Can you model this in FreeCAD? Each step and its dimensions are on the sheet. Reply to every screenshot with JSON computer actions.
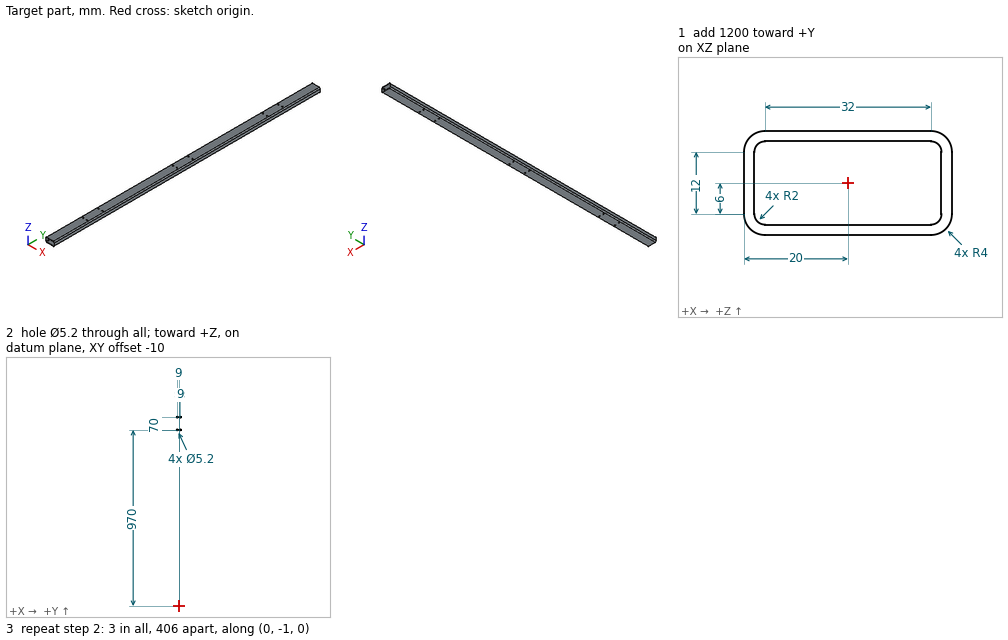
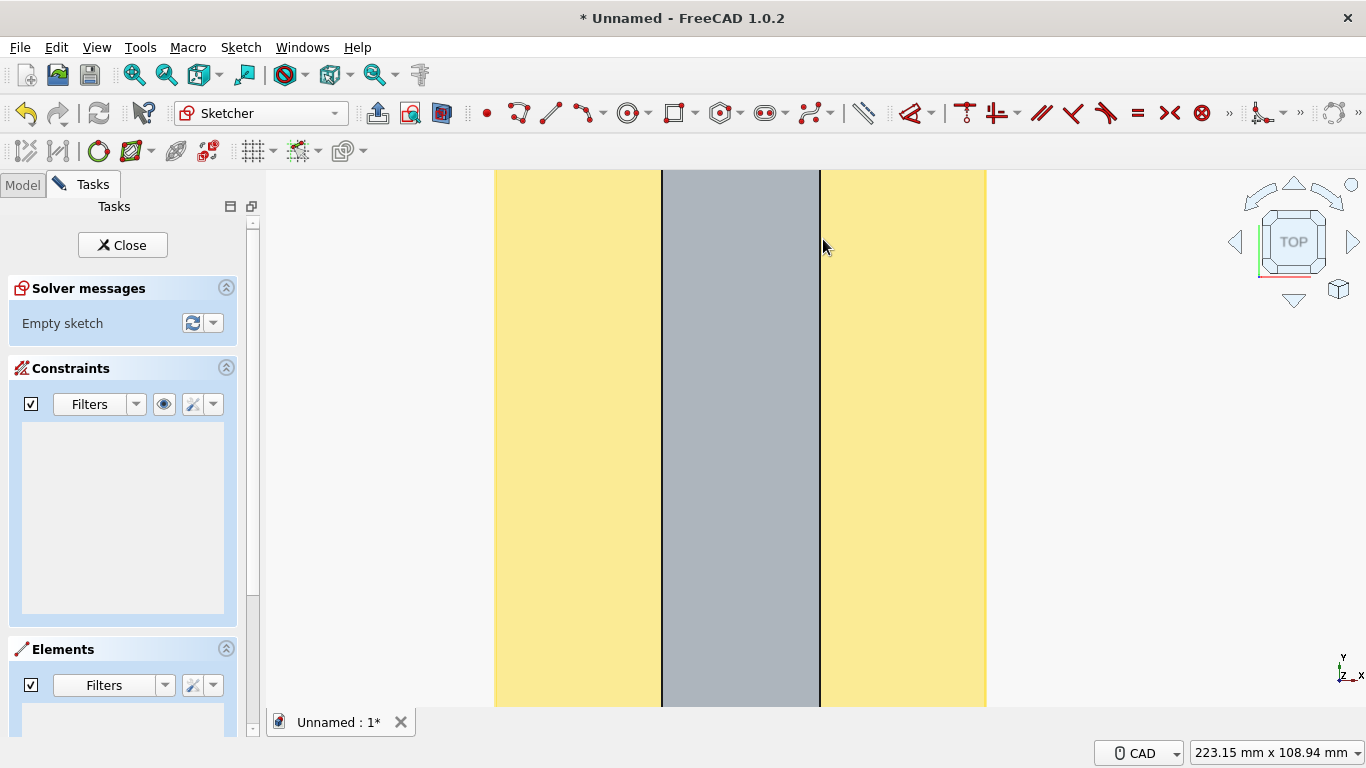
{"action": "left_click", "coordinate": [628, 114]}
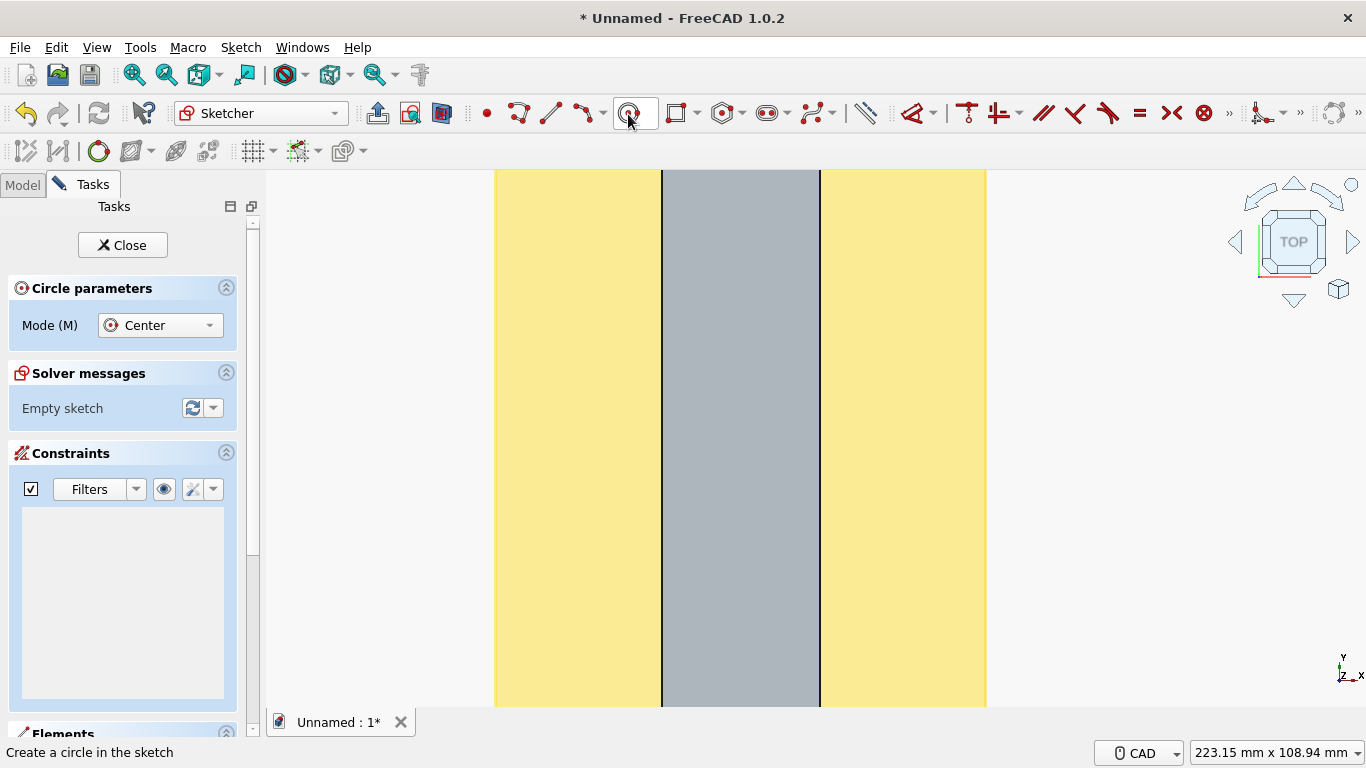
{"action": "scroll", "coordinate": [785, 268], "scroll_direction": "up", "scroll_amount": 3}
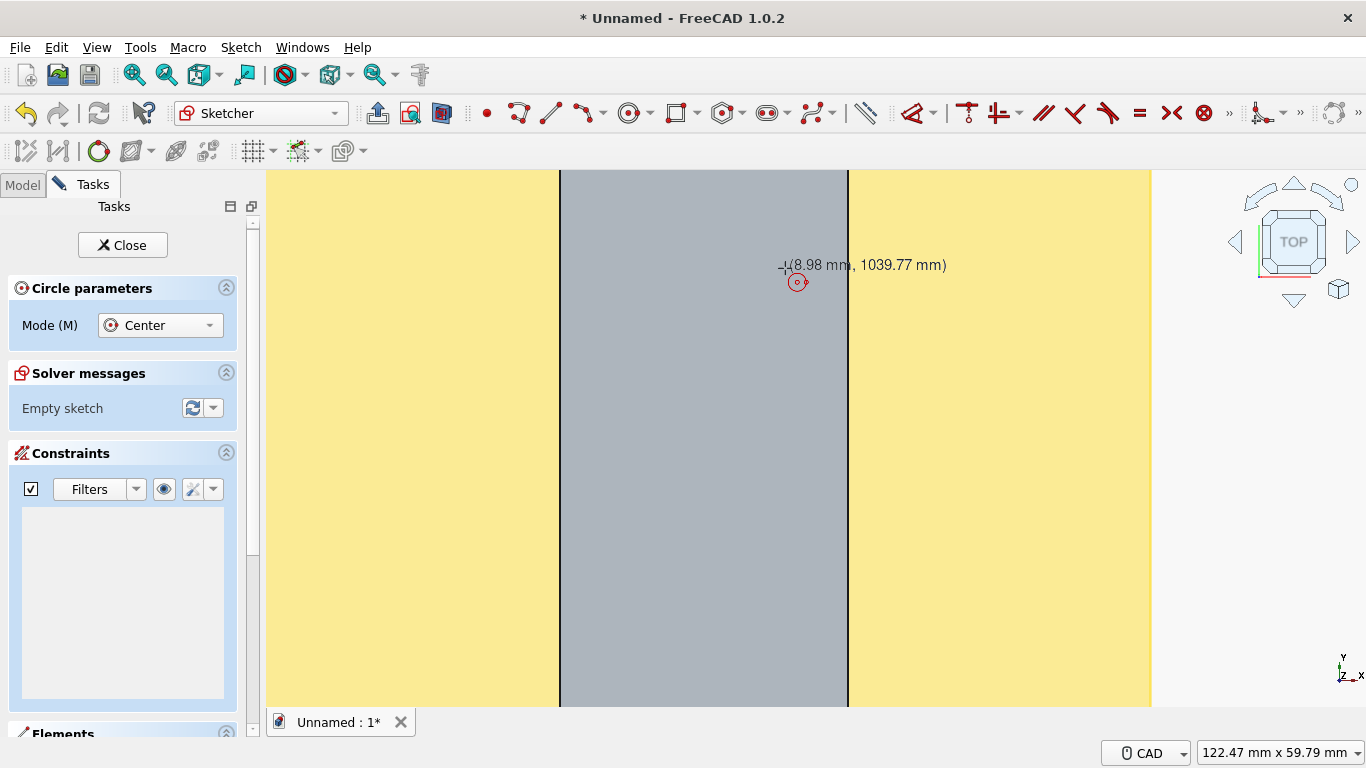
{"action": "left_click", "coordinate": [785, 268]}
{"action": "left_click", "coordinate": [801, 251]}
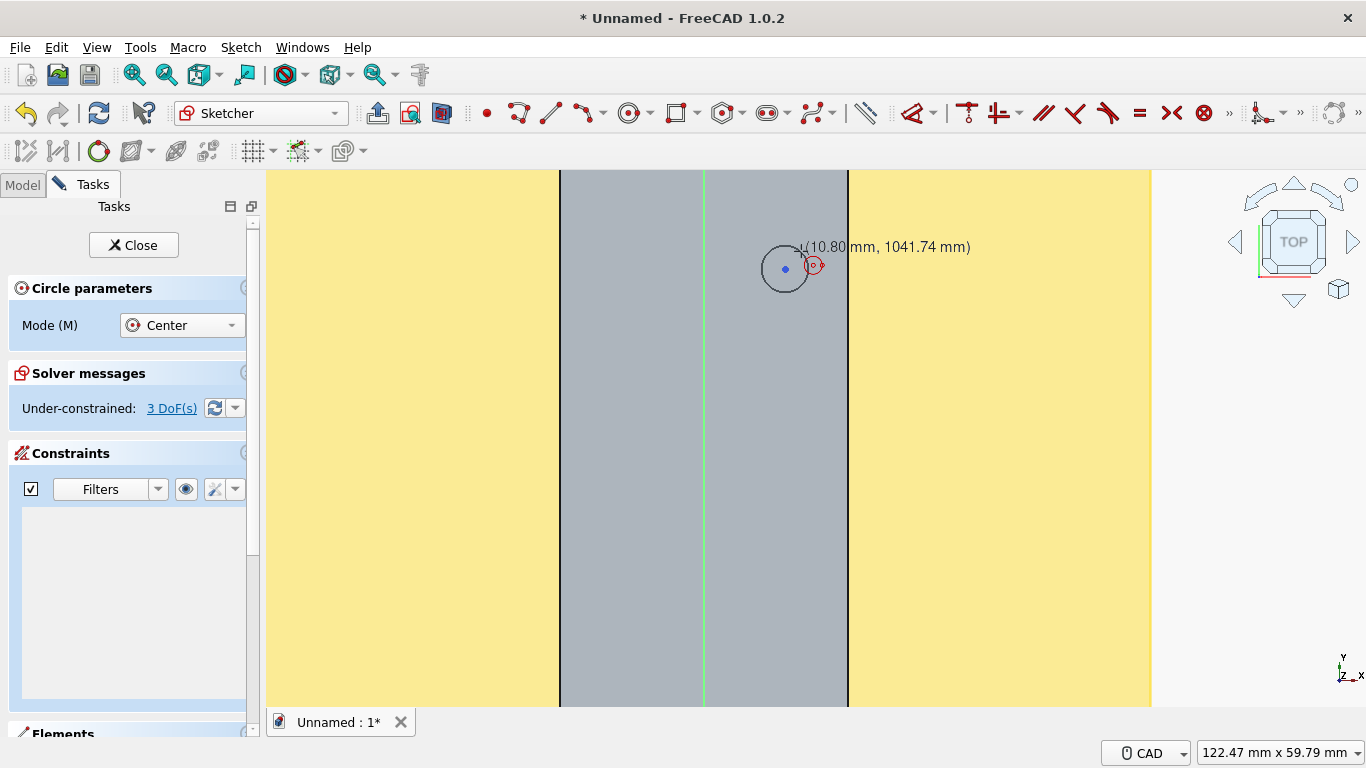
{"action": "left_click", "coordinate": [623, 268]}
{"action": "left_click", "coordinate": [640, 251]}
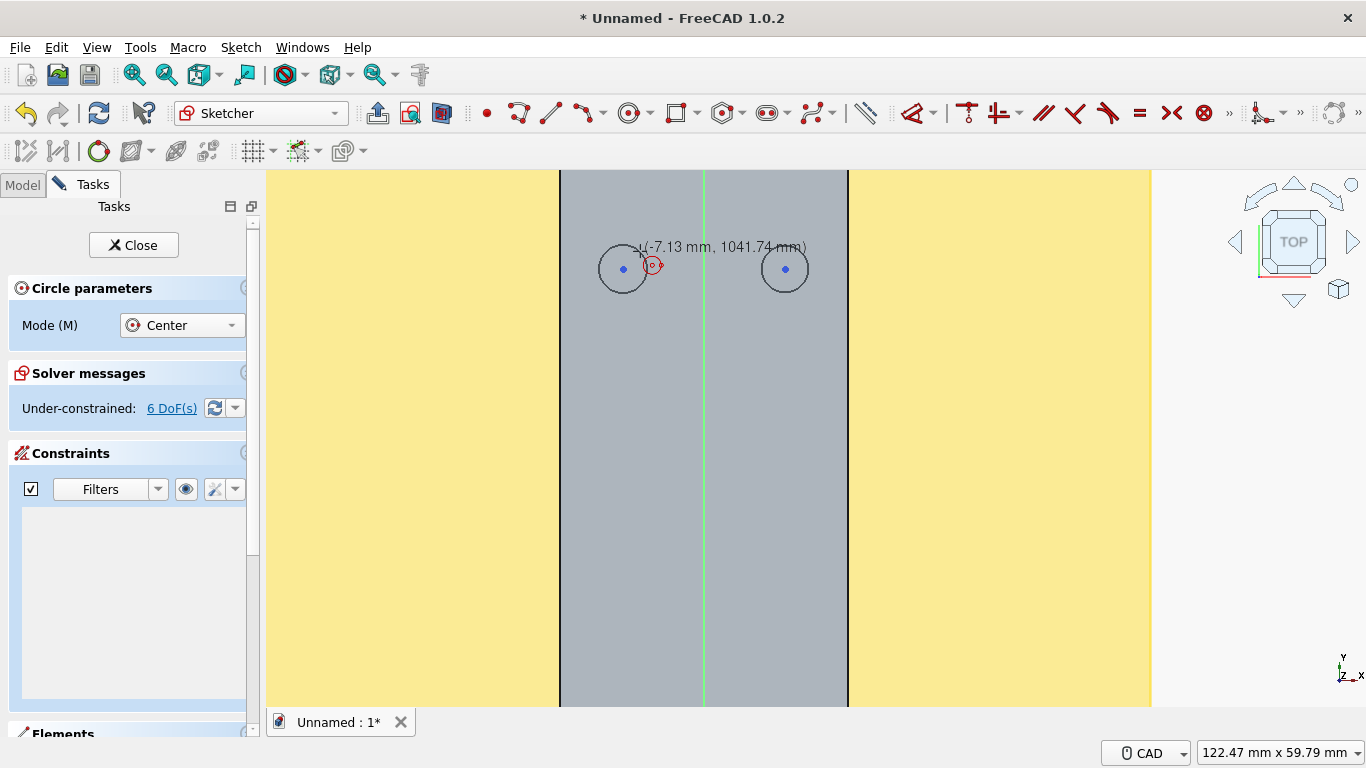
{"action": "scroll", "coordinate": [800, 264], "scroll_direction": "down", "scroll_amount": 3}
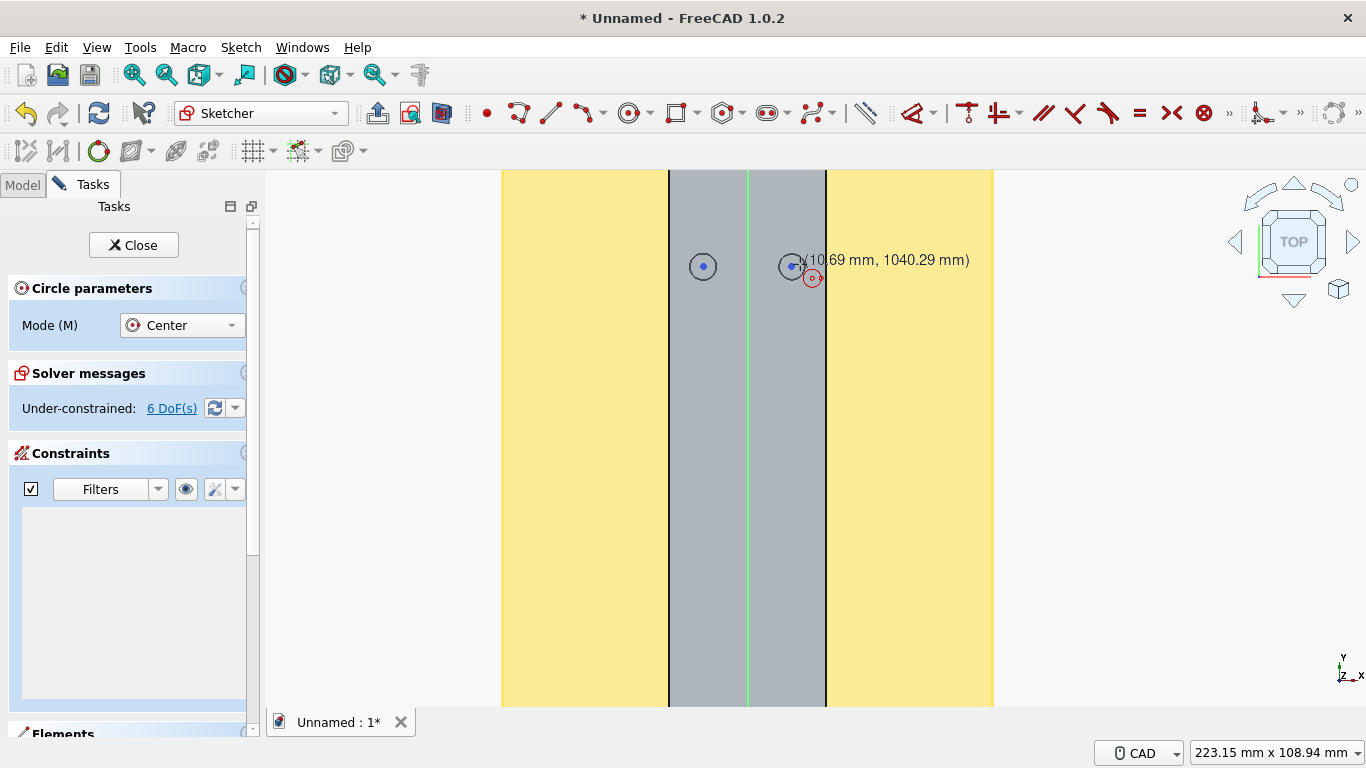
{"action": "scroll", "coordinate": [703, 611], "scroll_direction": "up", "scroll_amount": 3}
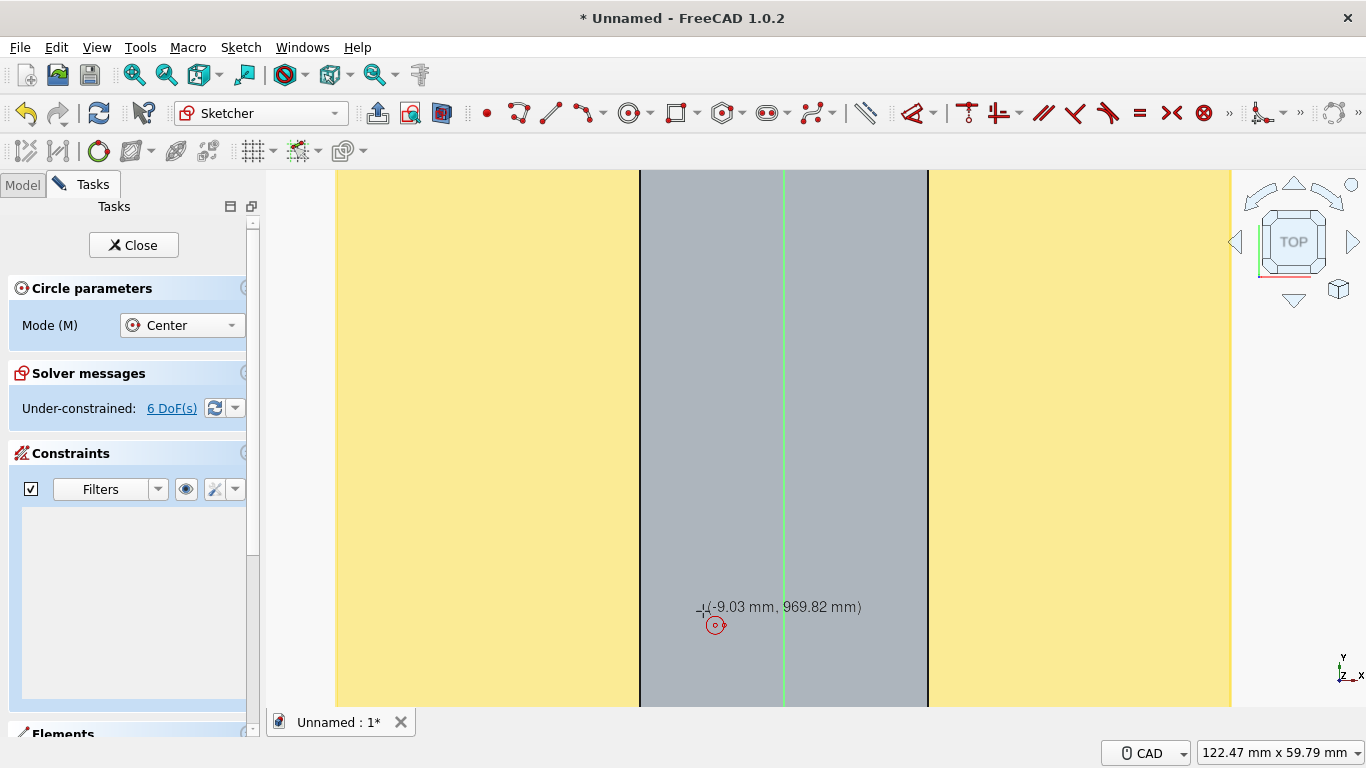
{"action": "left_click", "coordinate": [703, 611]}
{"action": "left_click", "coordinate": [719, 594]}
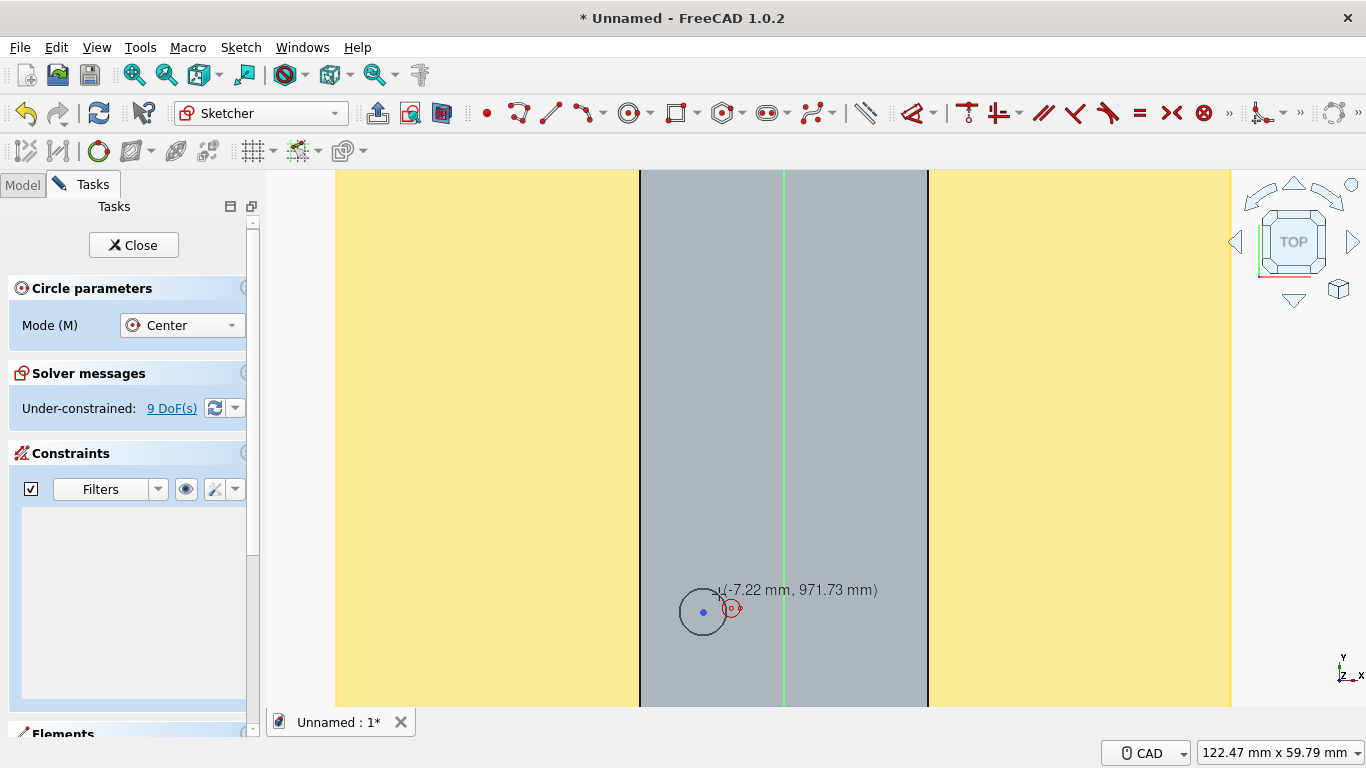
{"action": "left_click", "coordinate": [865, 611]}
{"action": "left_click", "coordinate": [881, 594]}
{"action": "key", "text": "Escape"}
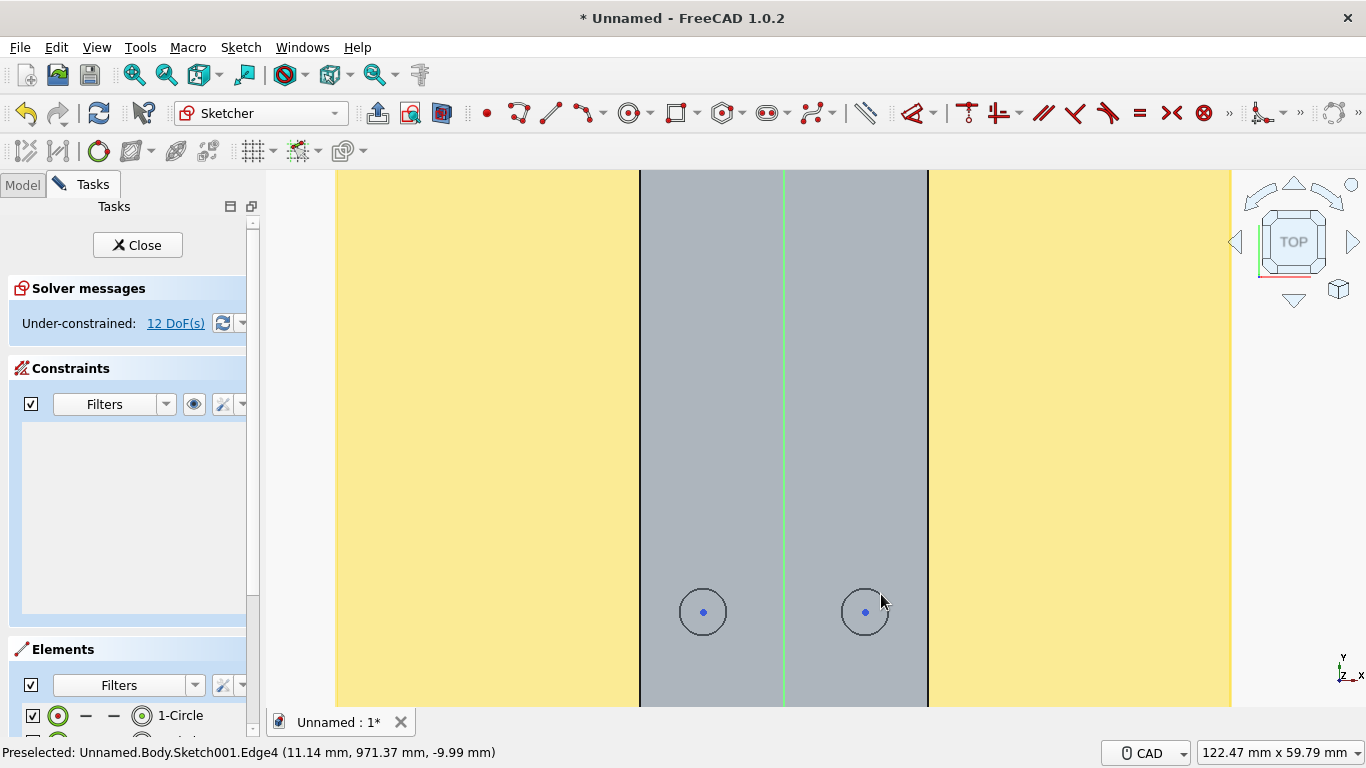
{"action": "scroll", "coordinate": [703, 612], "scroll_direction": "down", "scroll_amount": 3}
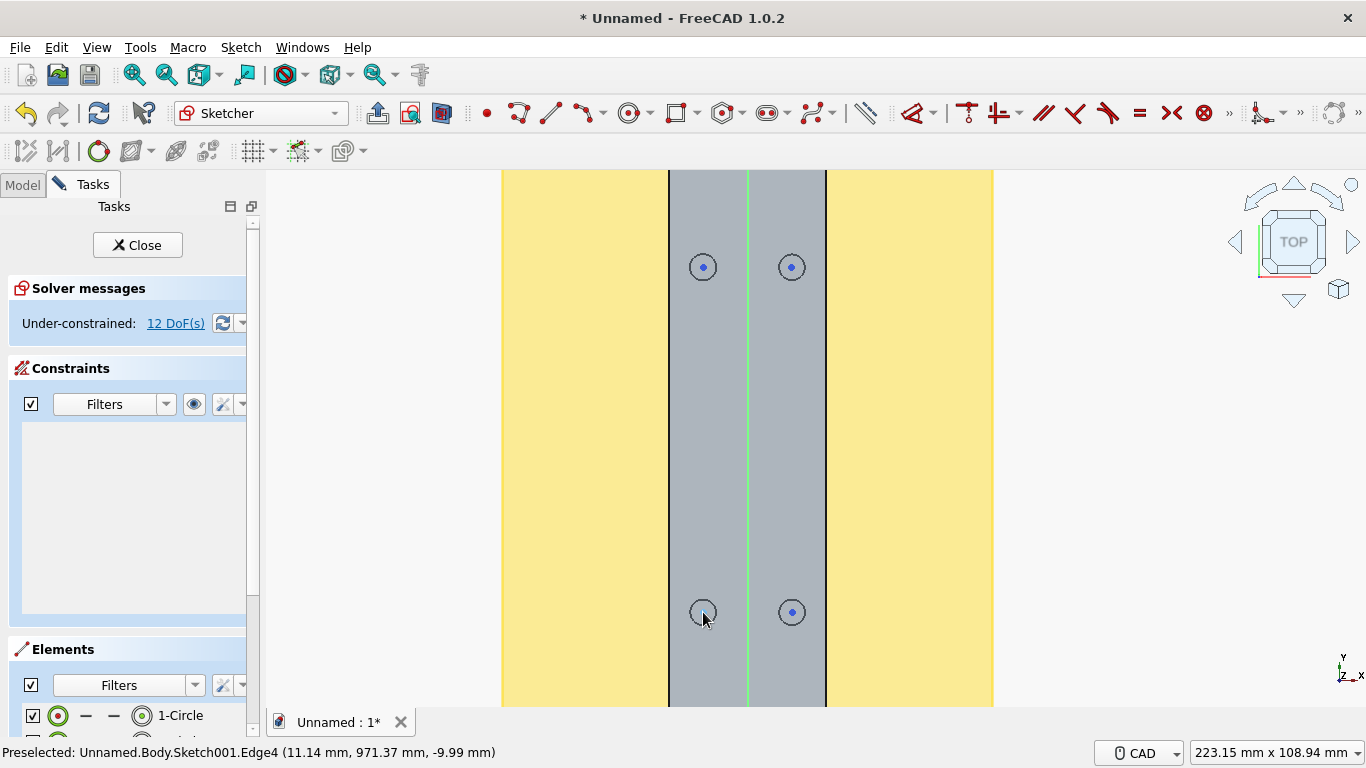
{"action": "left_click", "coordinate": [801, 258]}